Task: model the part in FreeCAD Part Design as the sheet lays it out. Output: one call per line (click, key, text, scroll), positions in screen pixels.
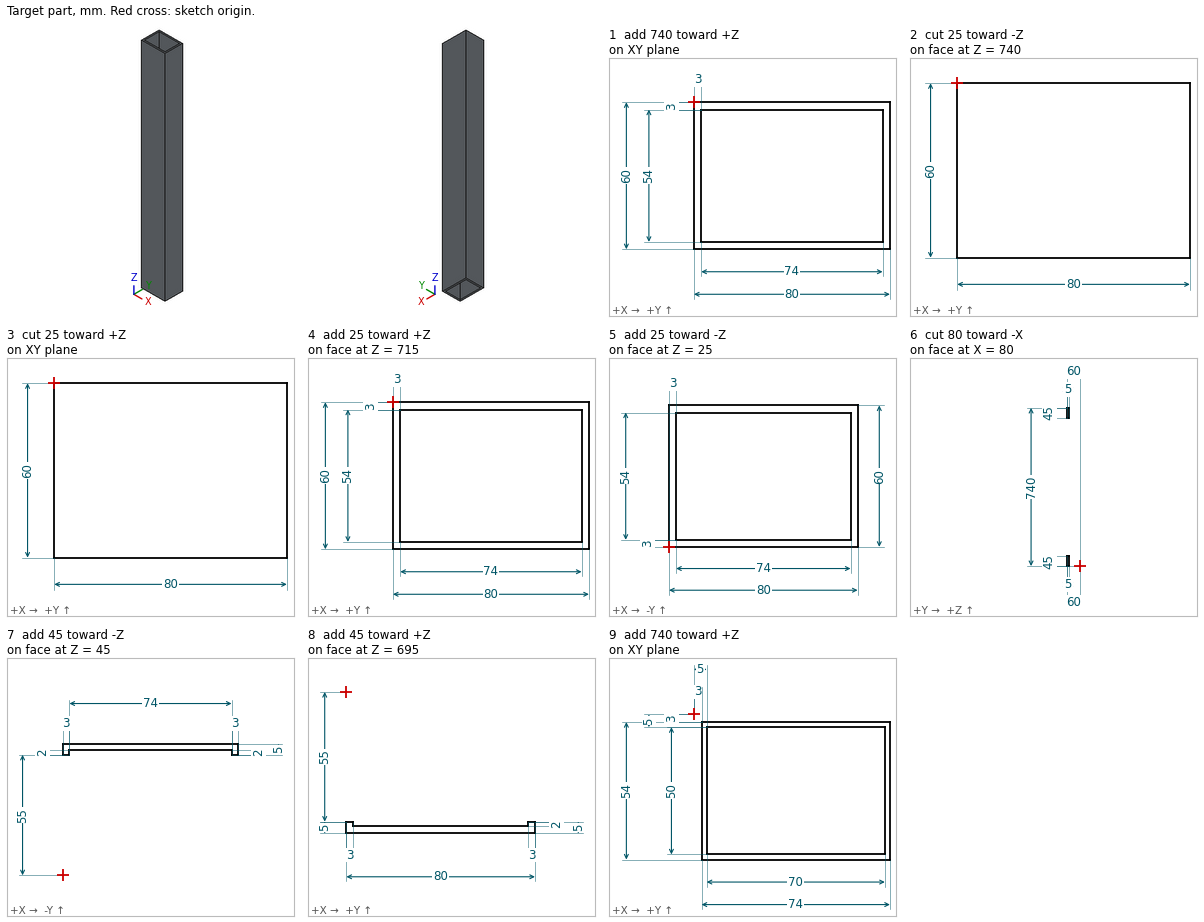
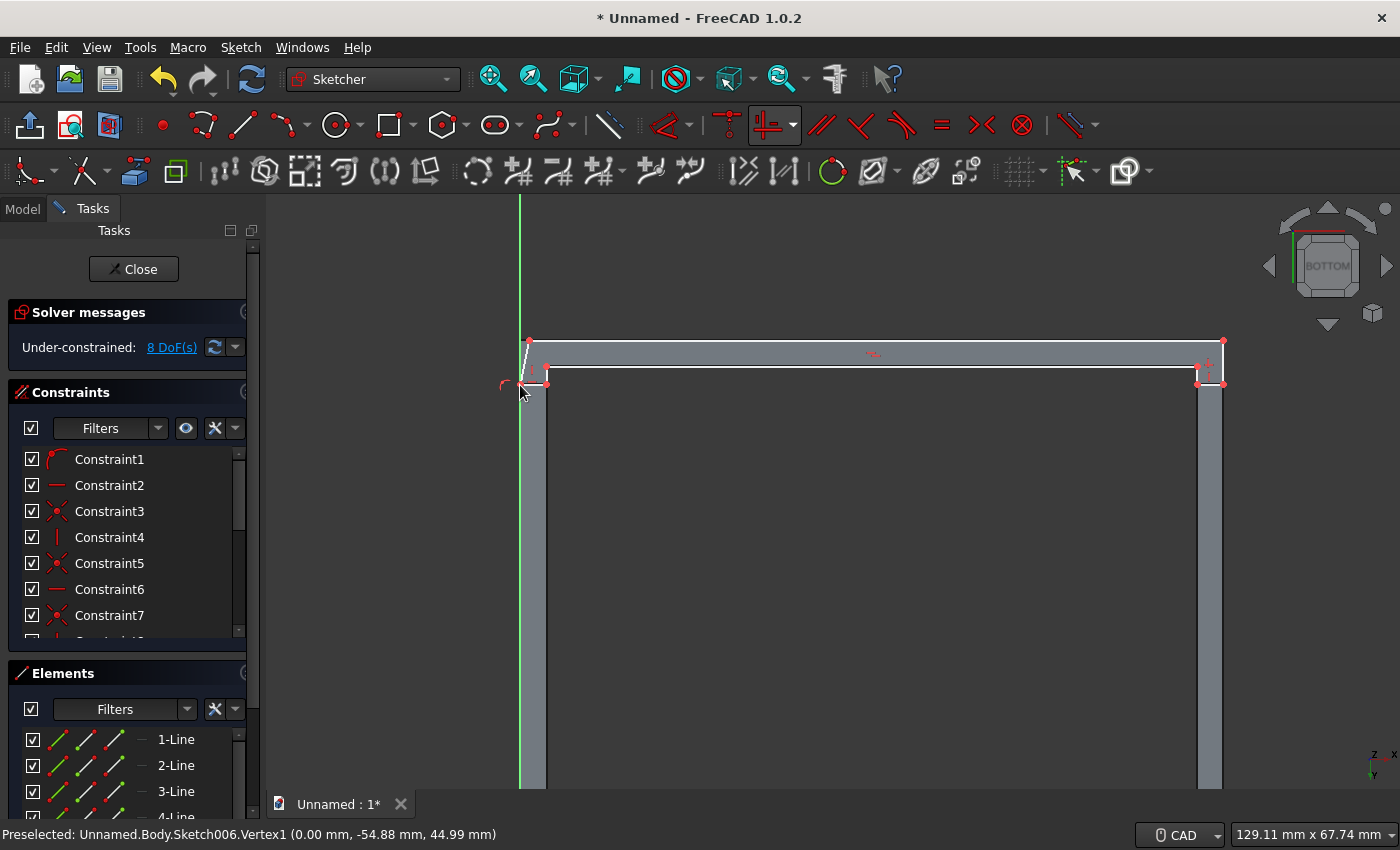
click(523, 372)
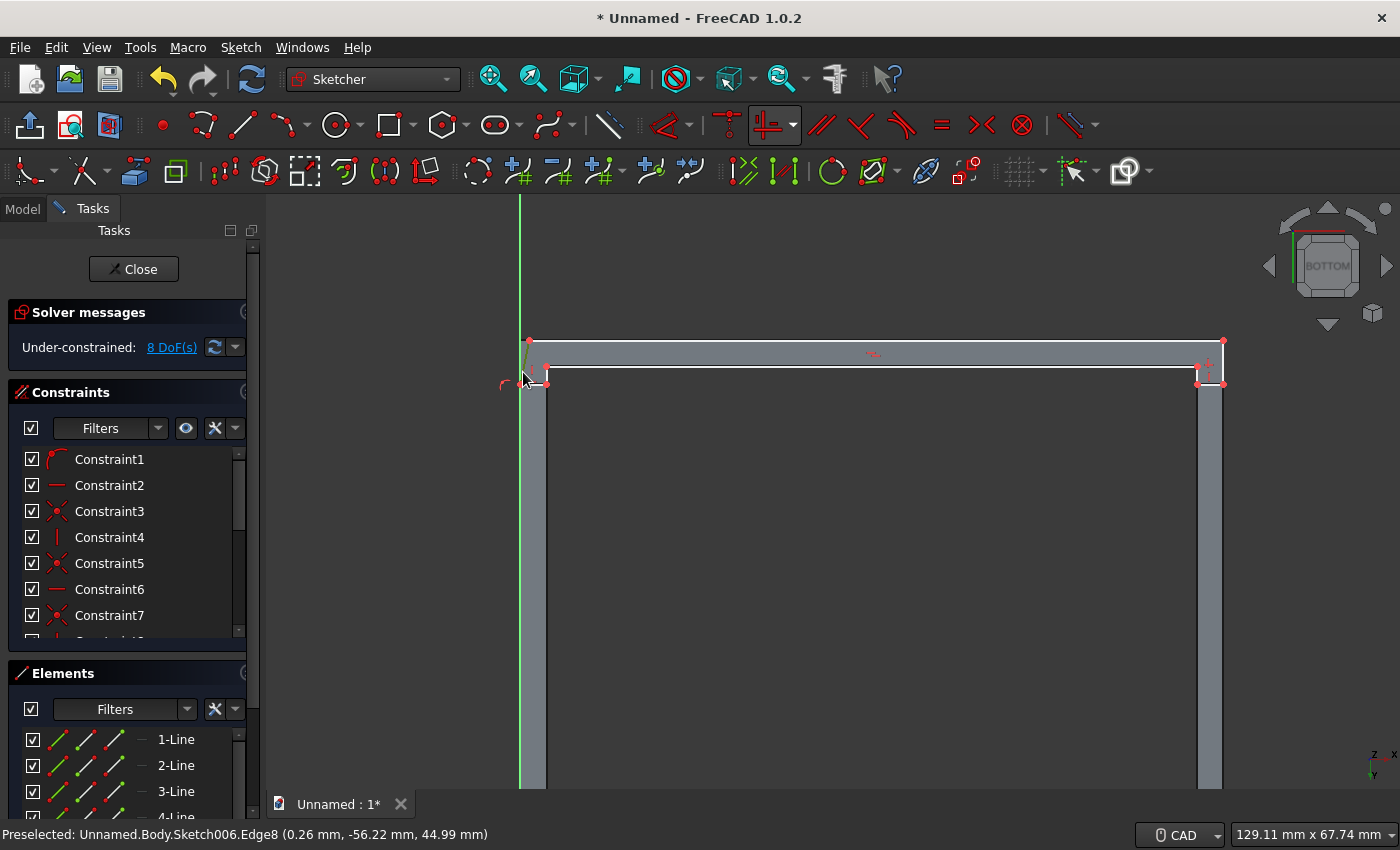
click(796, 126)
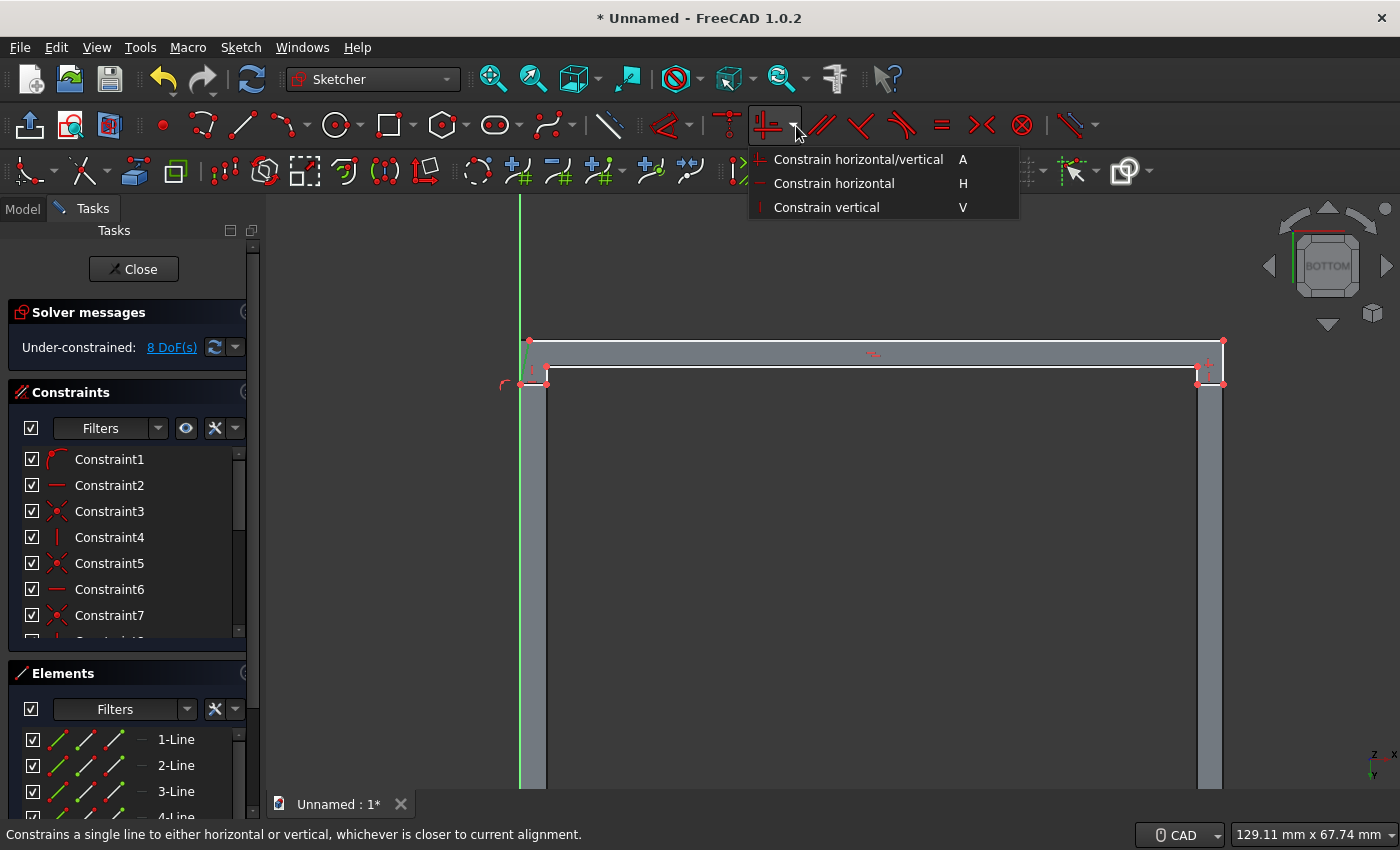
click(884, 207)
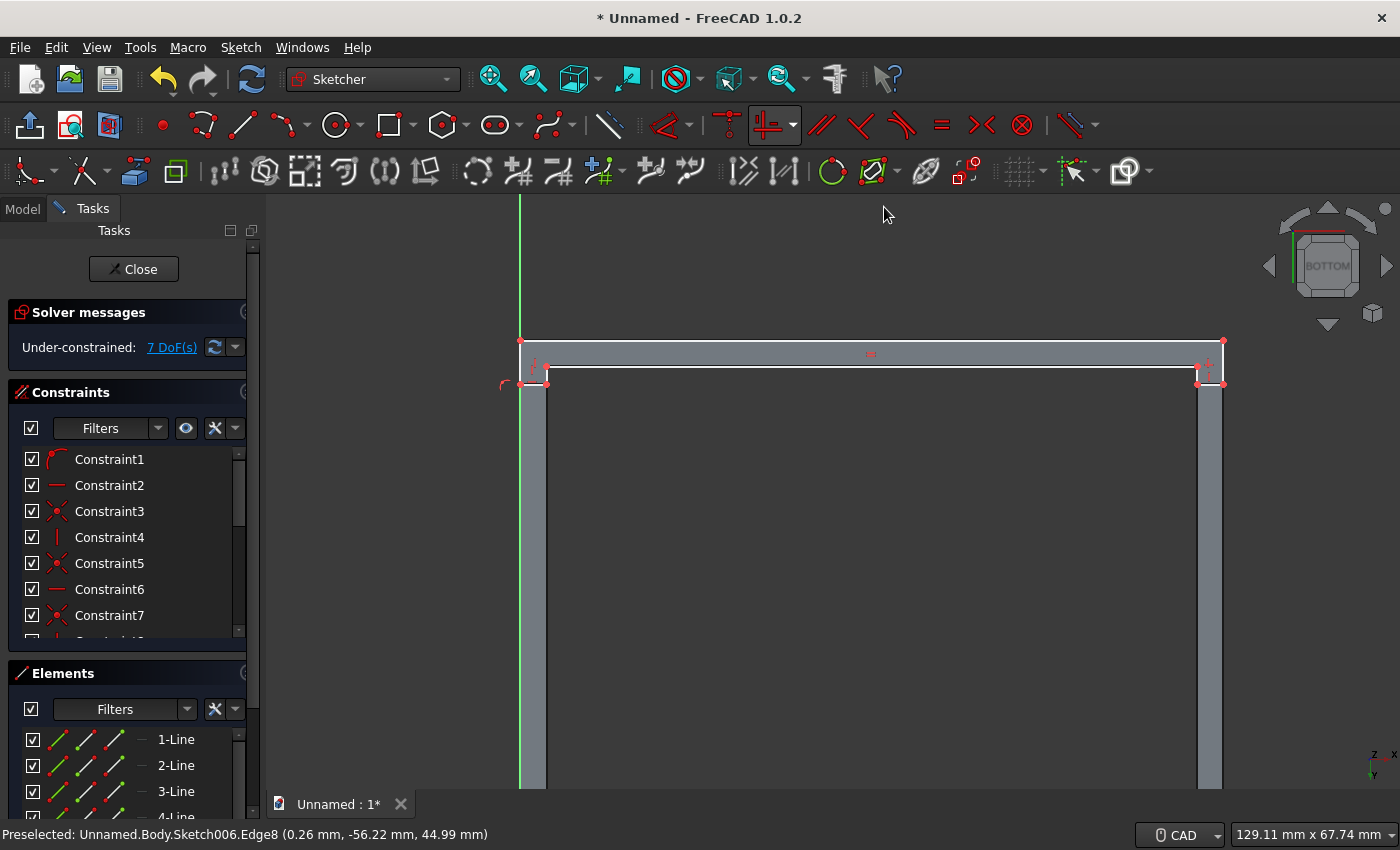
key(d)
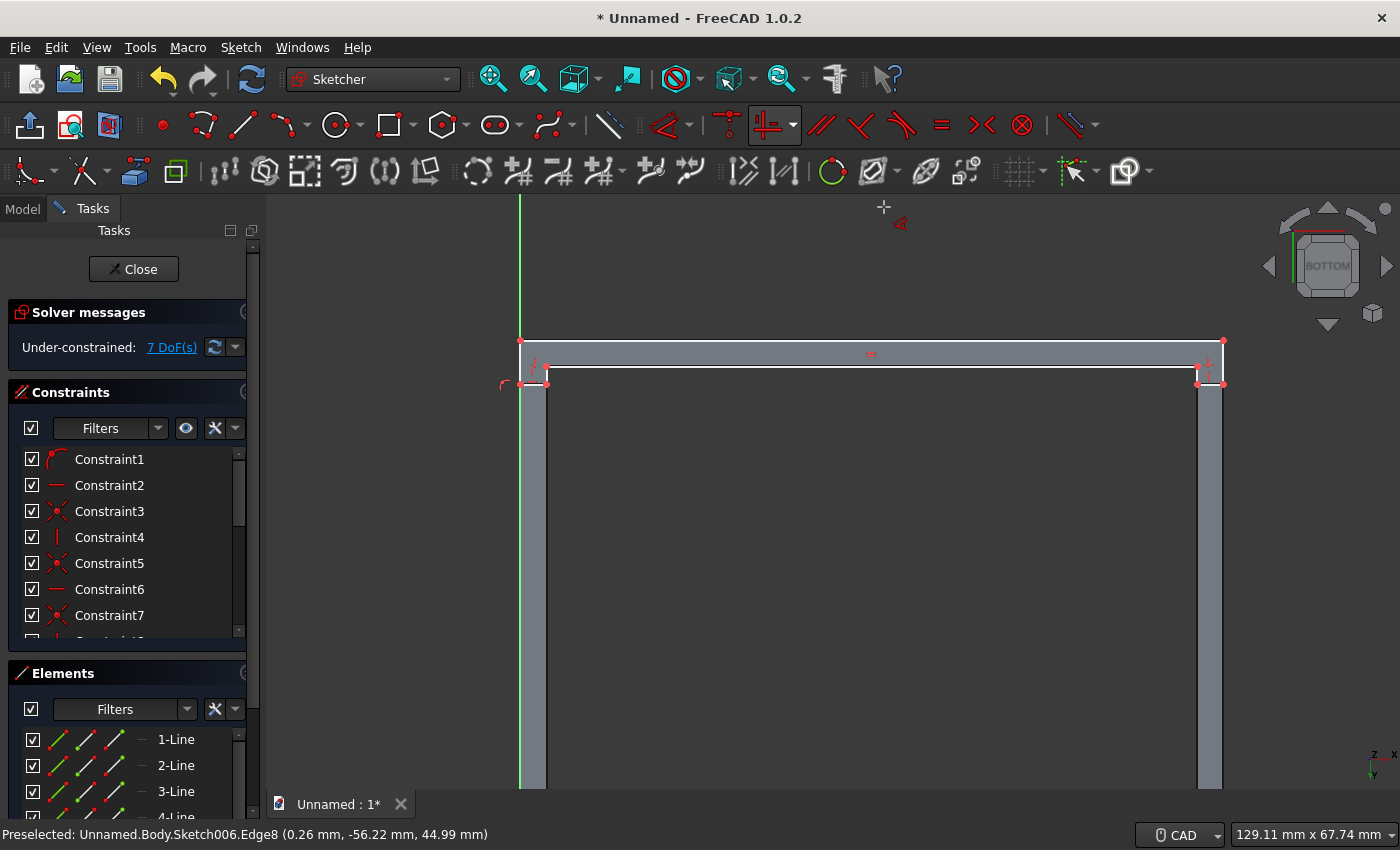
scroll(531, 385, up, 3)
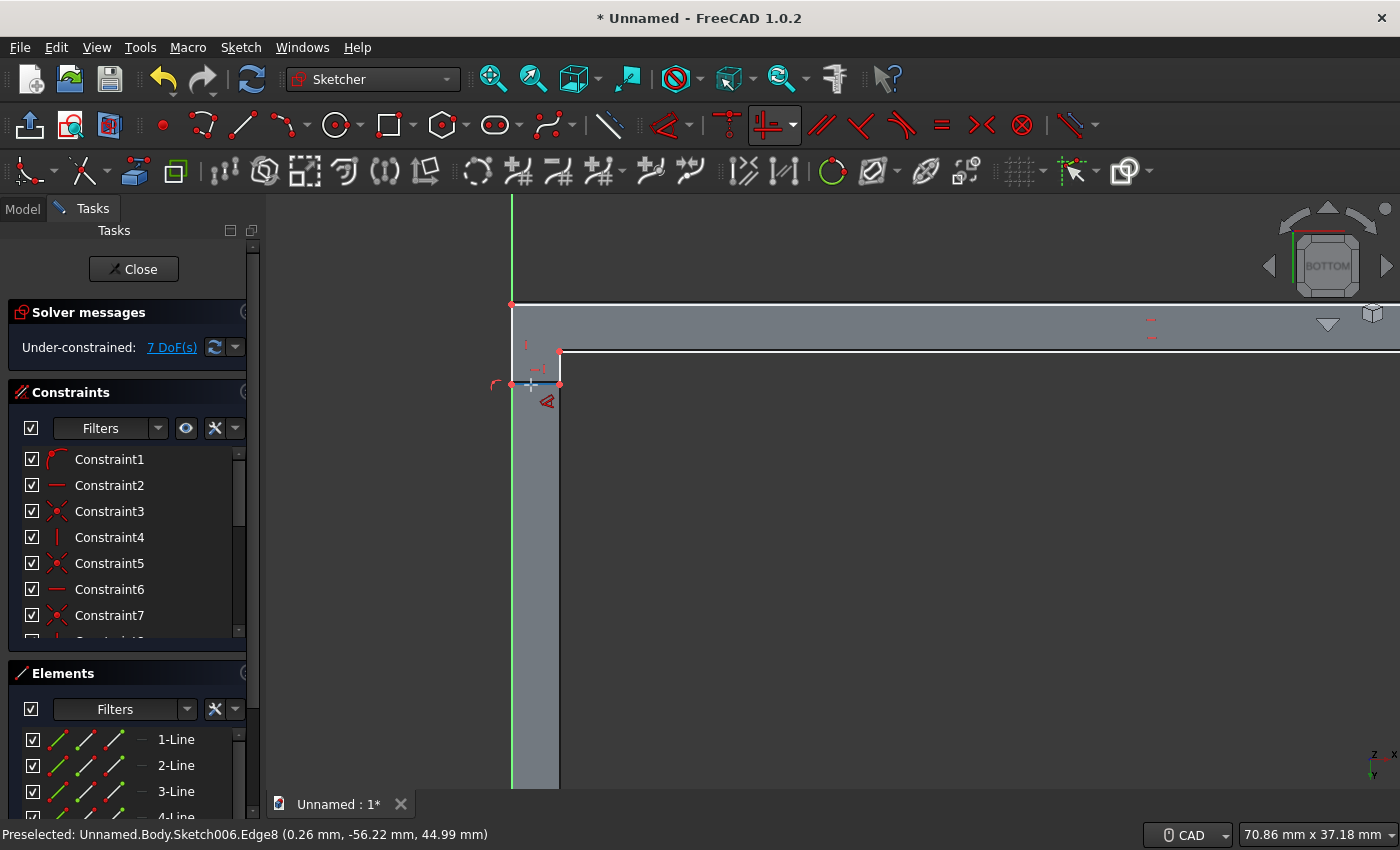
click(531, 384)
click(536, 350)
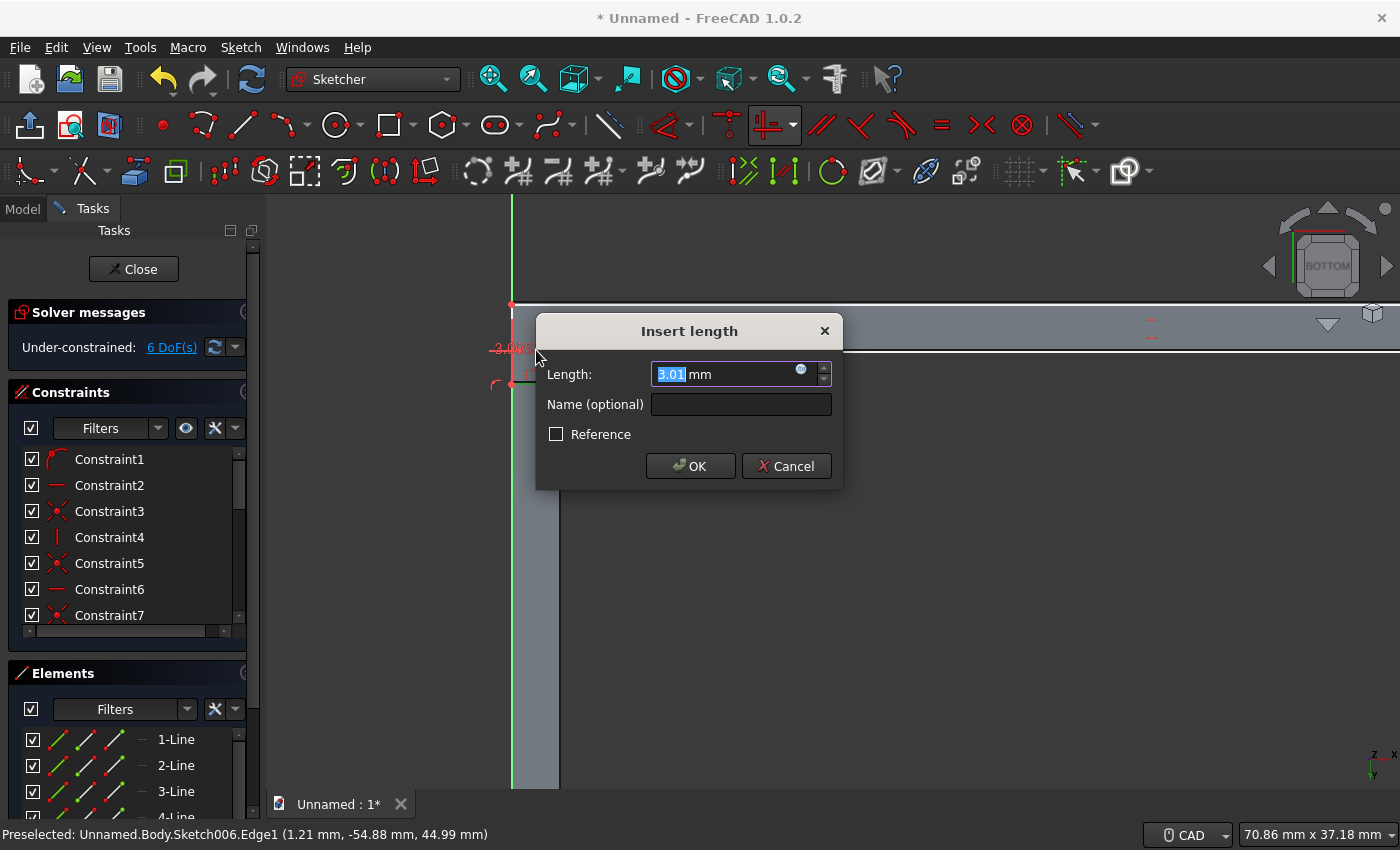
text(3)
key(Return)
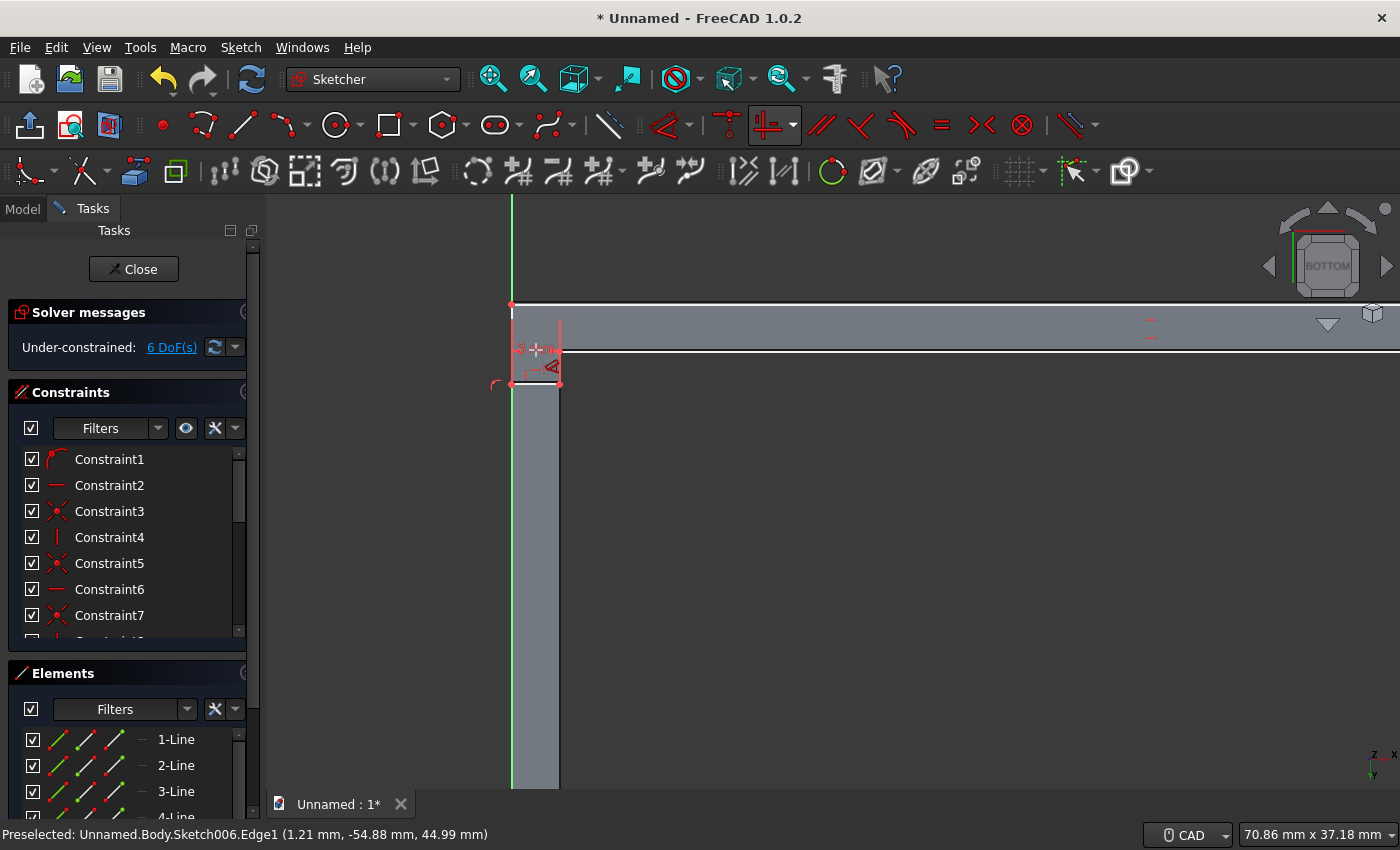
scroll(560, 375, up, 2)